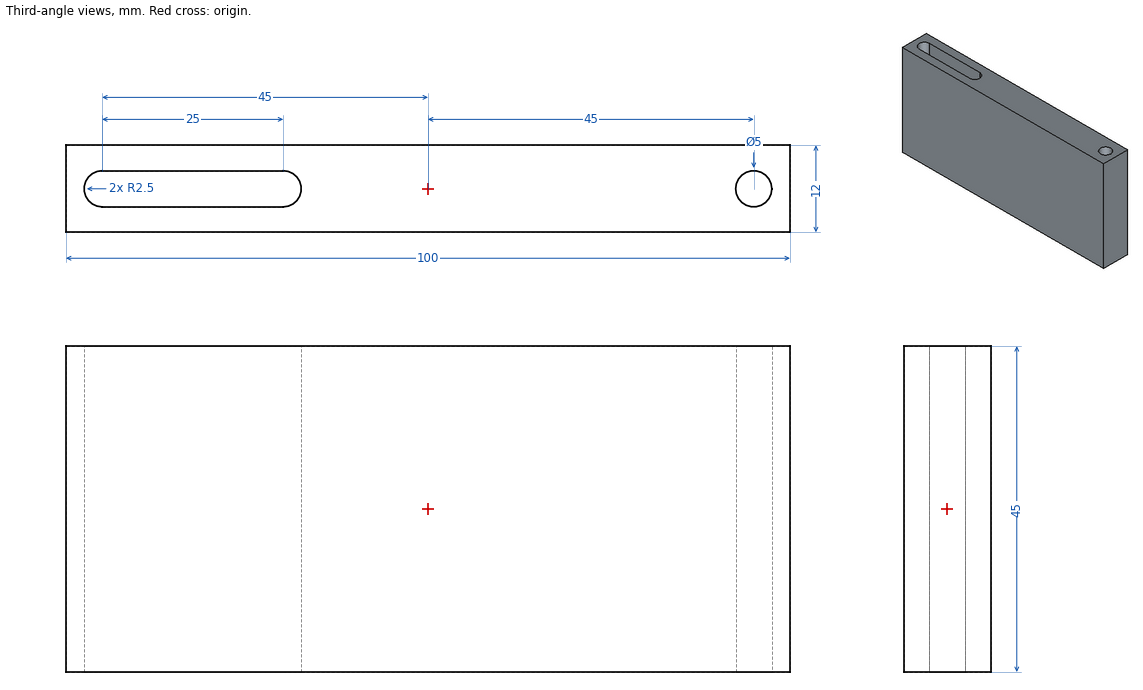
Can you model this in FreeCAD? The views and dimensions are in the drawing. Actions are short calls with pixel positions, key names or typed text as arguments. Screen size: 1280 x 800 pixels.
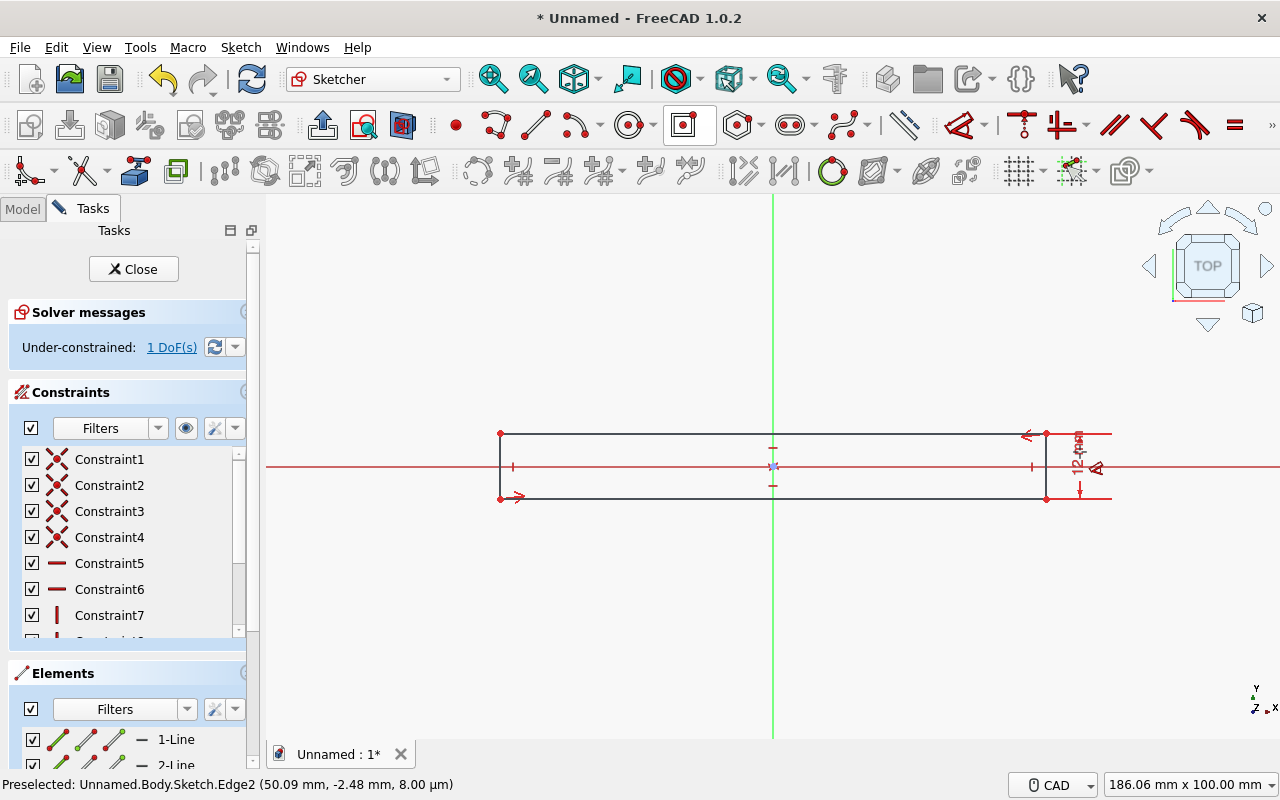
click(664, 499)
click(647, 533)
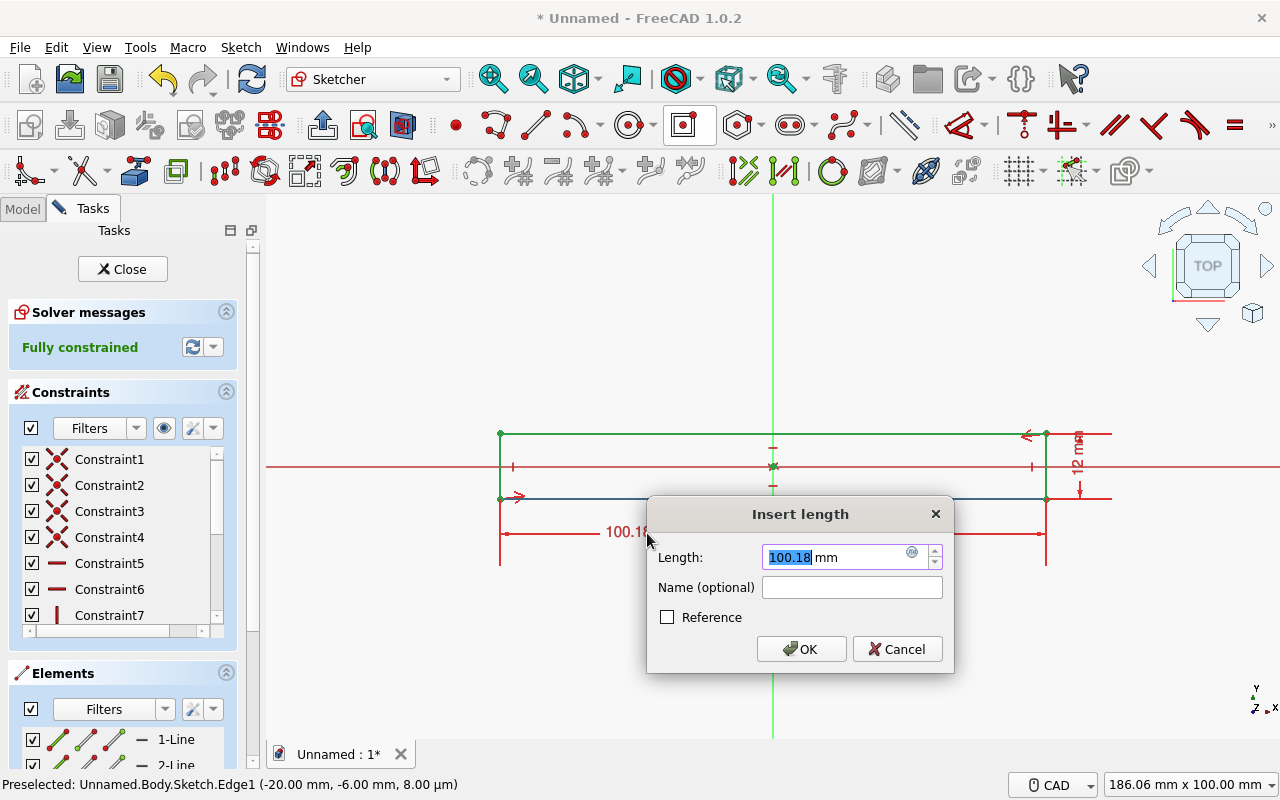
text(100)
key(Return)
key(Escape)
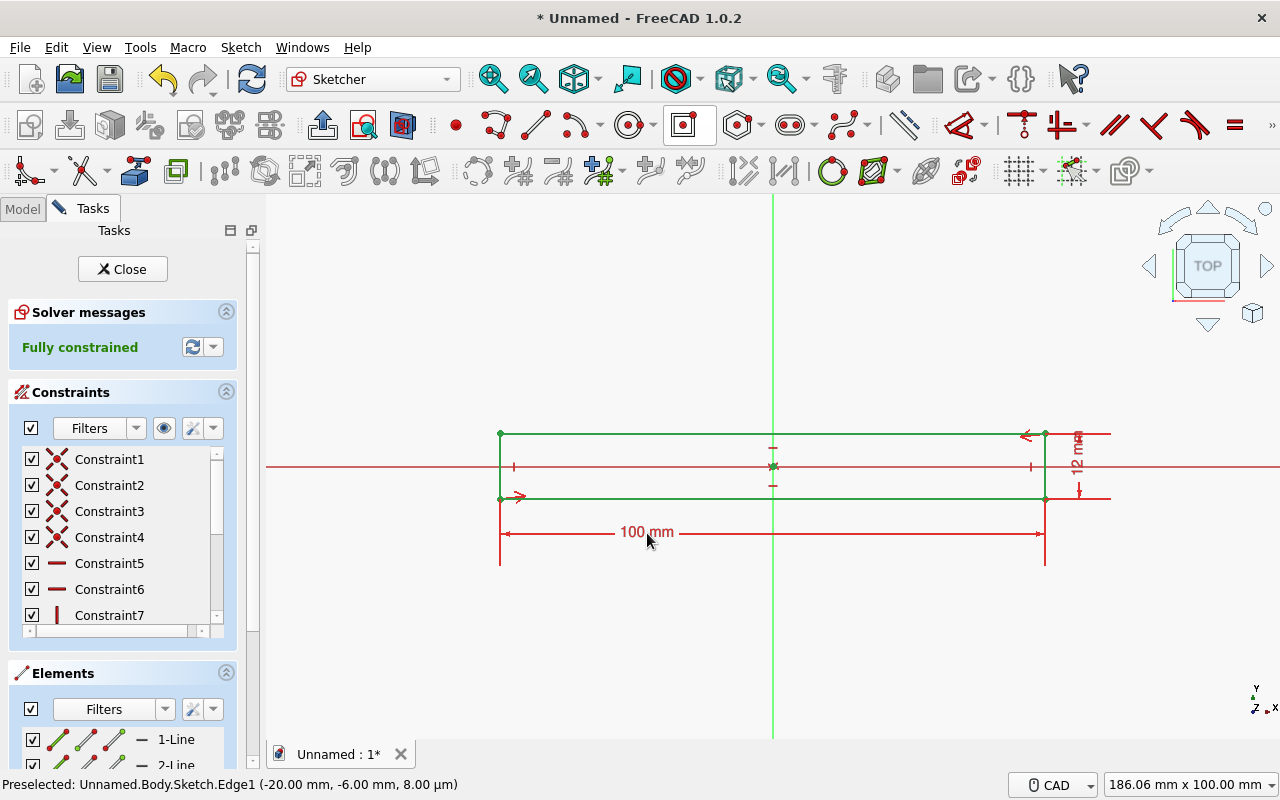
click(123, 269)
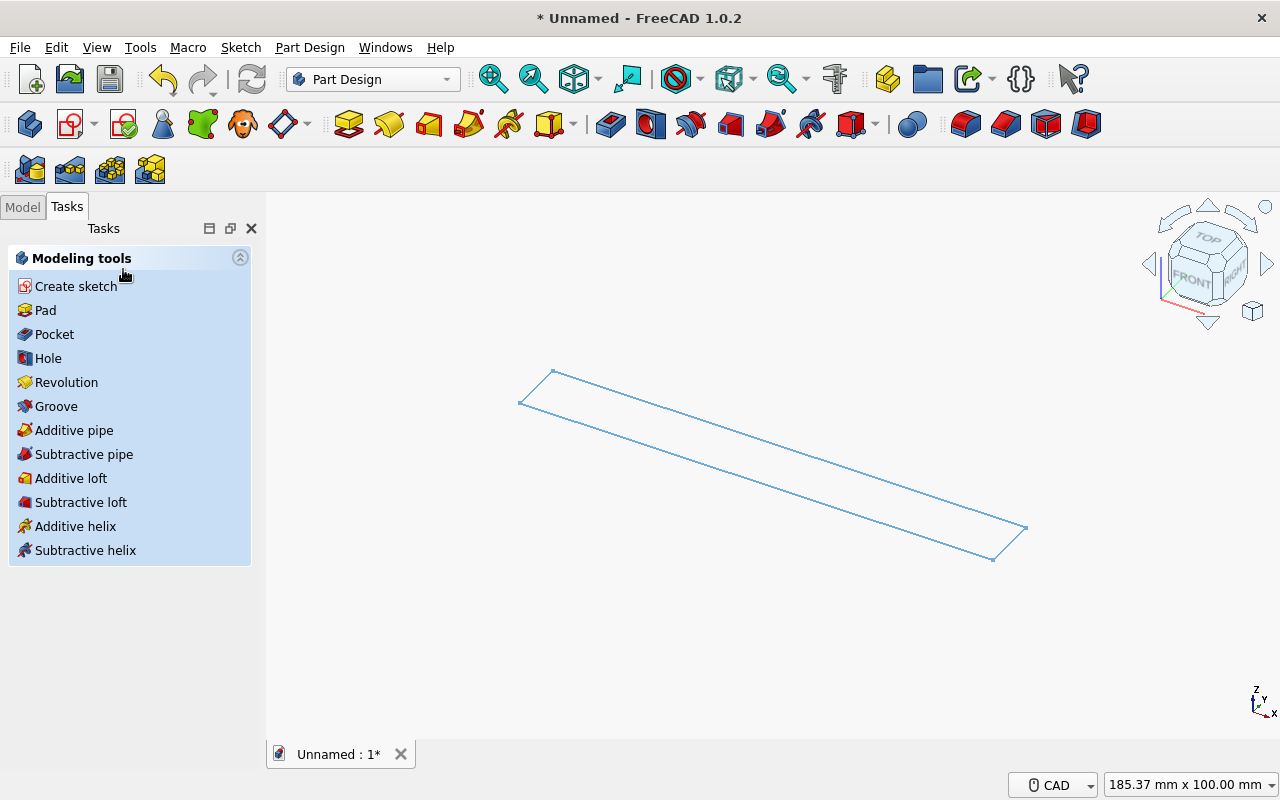
click(350, 124)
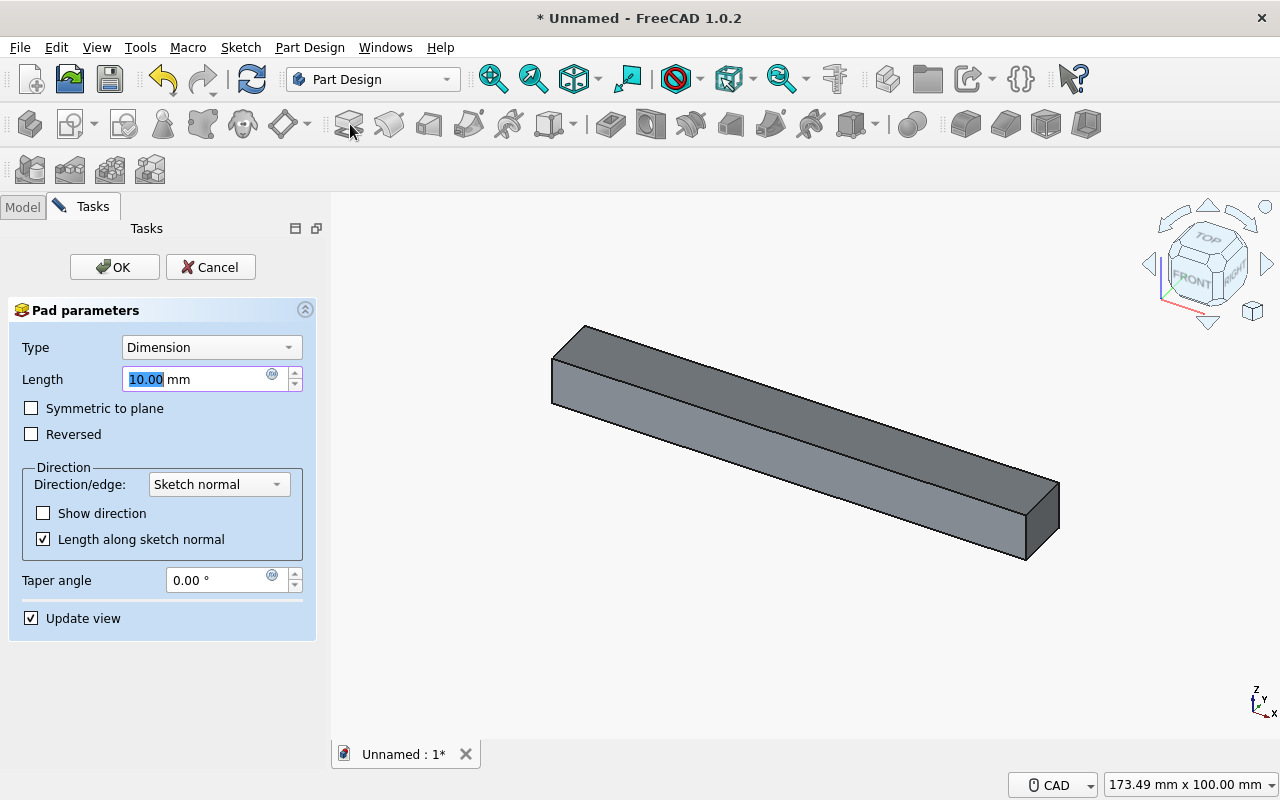
text(45)
key(Tab)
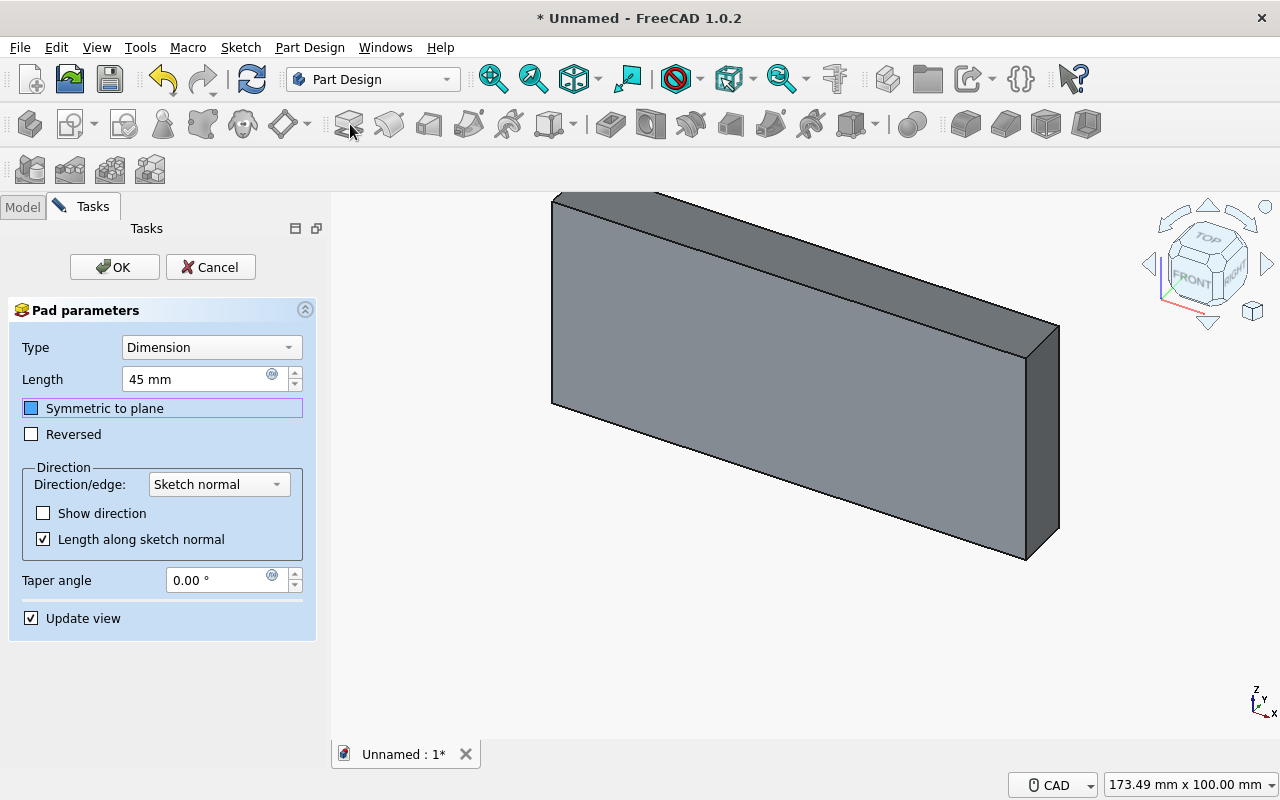
click(30, 408)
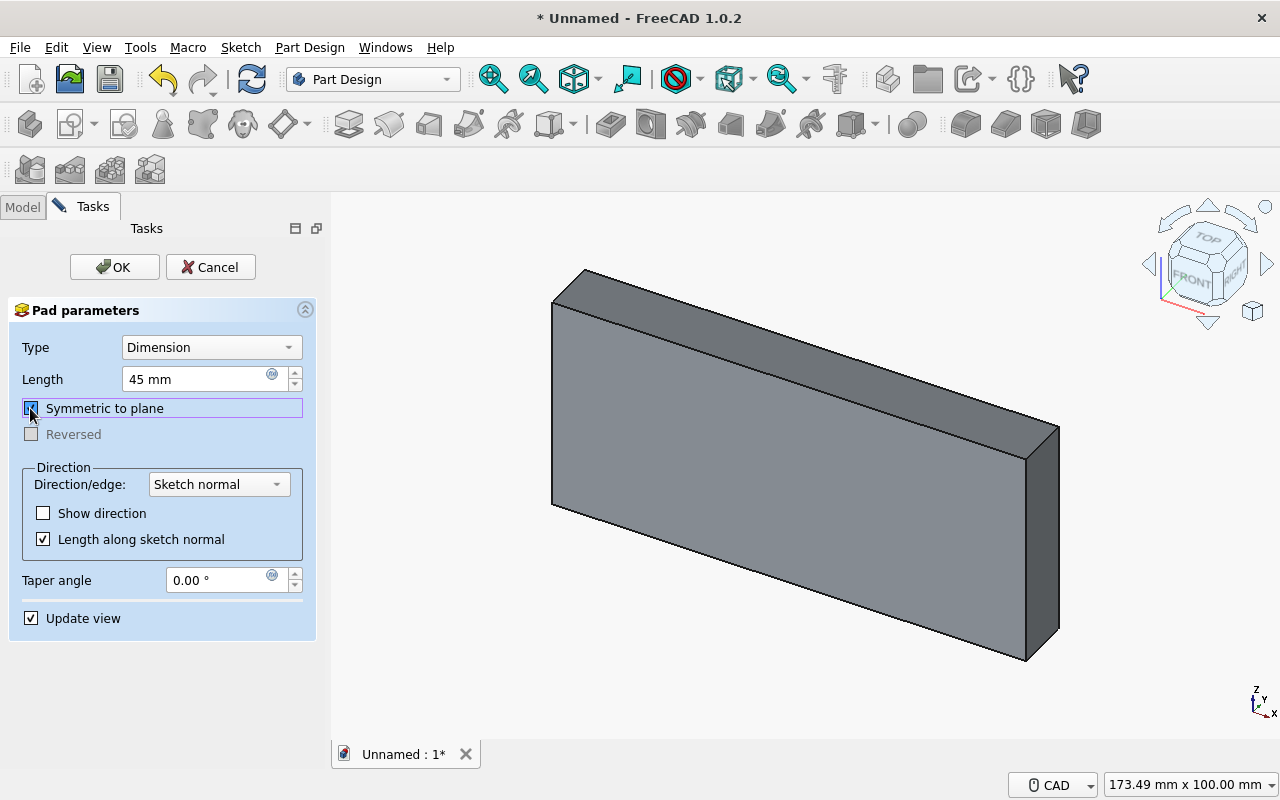
click(115, 267)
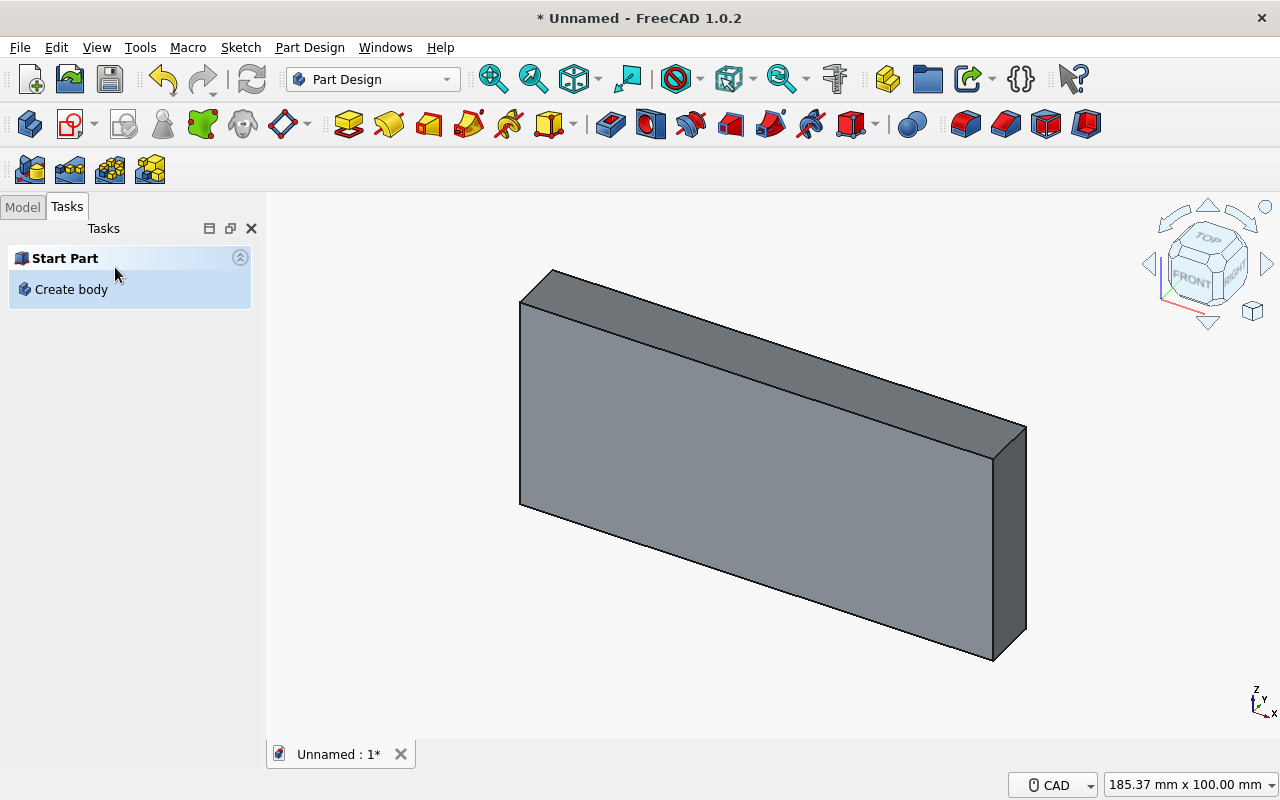
click(976, 431)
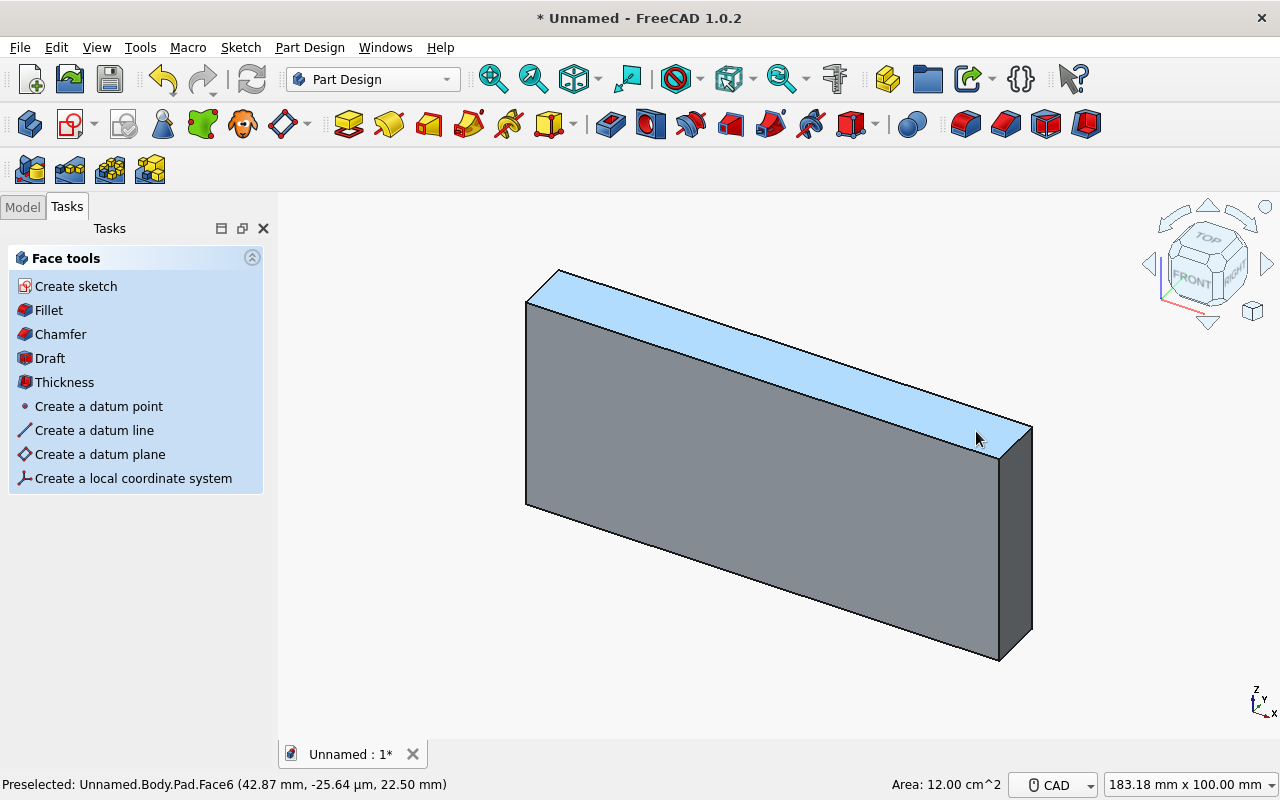
click(70, 124)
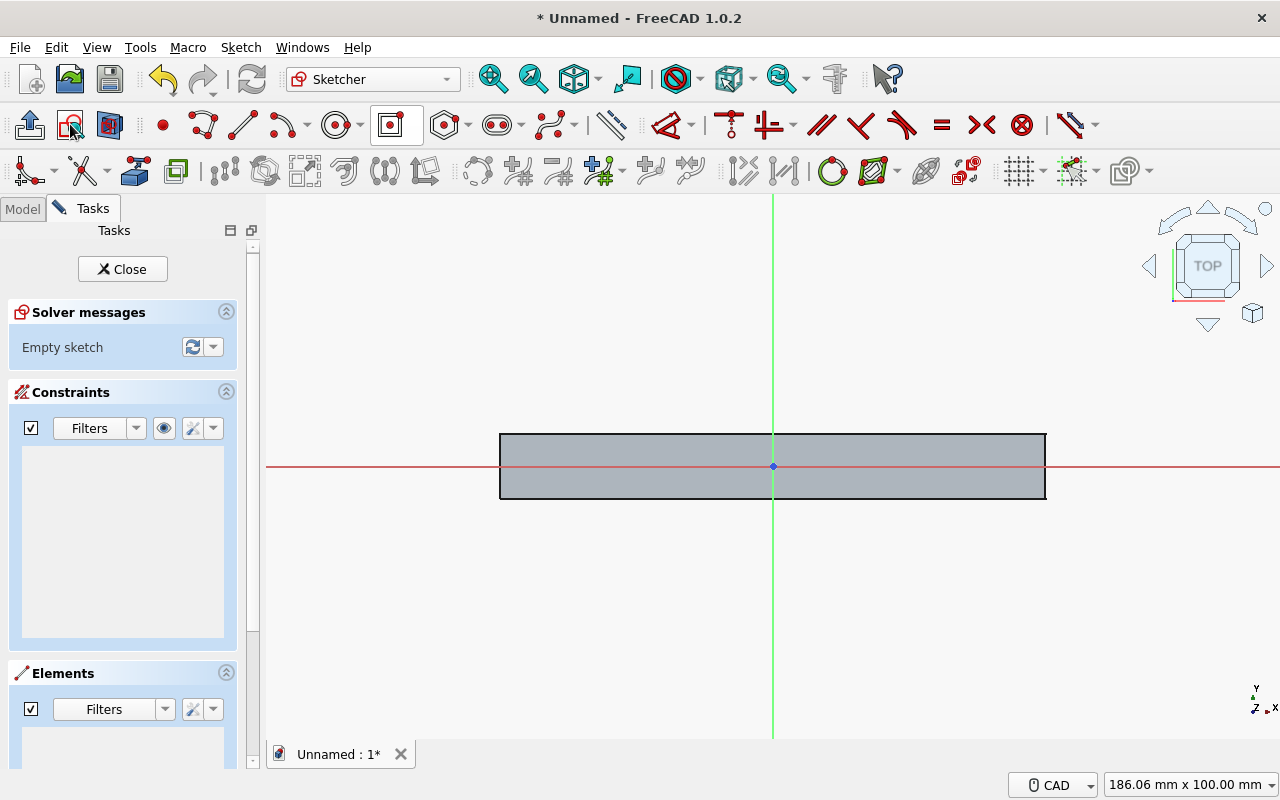
scroll(1043, 466, up, 13)